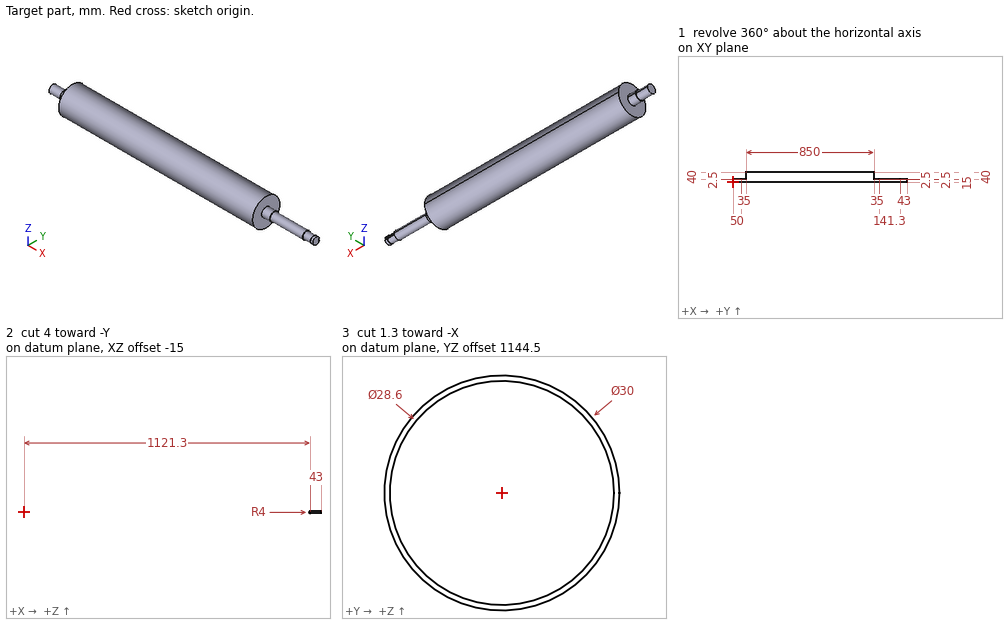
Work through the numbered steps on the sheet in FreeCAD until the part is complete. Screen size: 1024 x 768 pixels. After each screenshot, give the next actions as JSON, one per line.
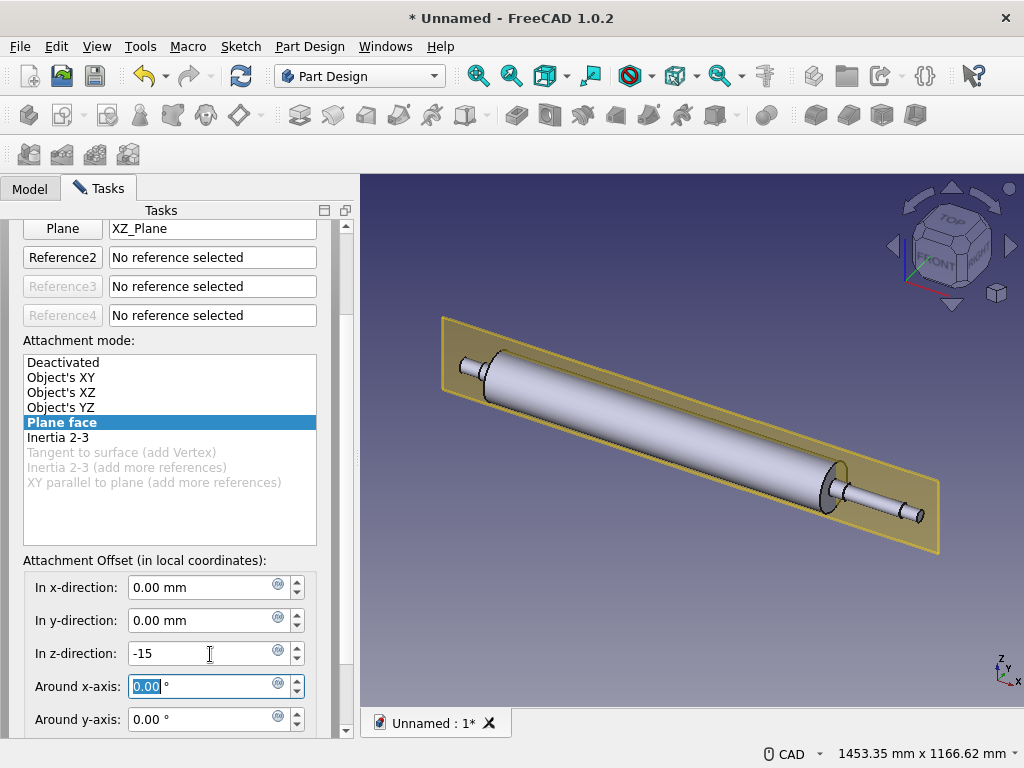
{"action": "scroll", "coordinate": [346, 479], "scroll_direction": "up", "scroll_amount": 3}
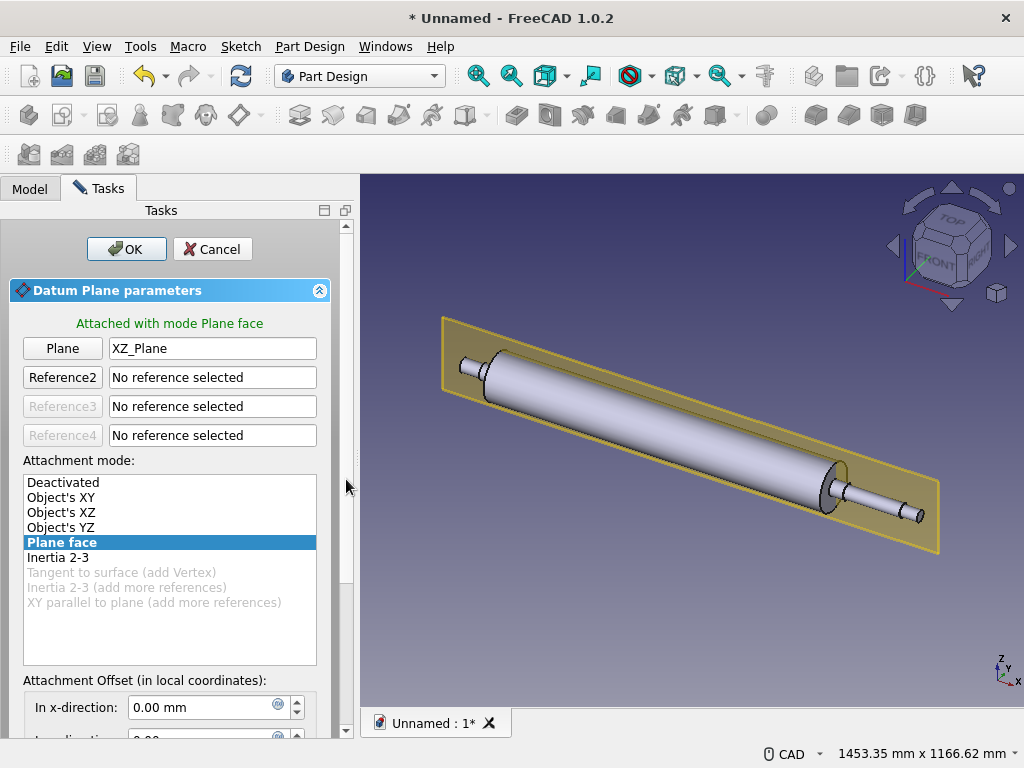
{"action": "left_click", "coordinate": [127, 249]}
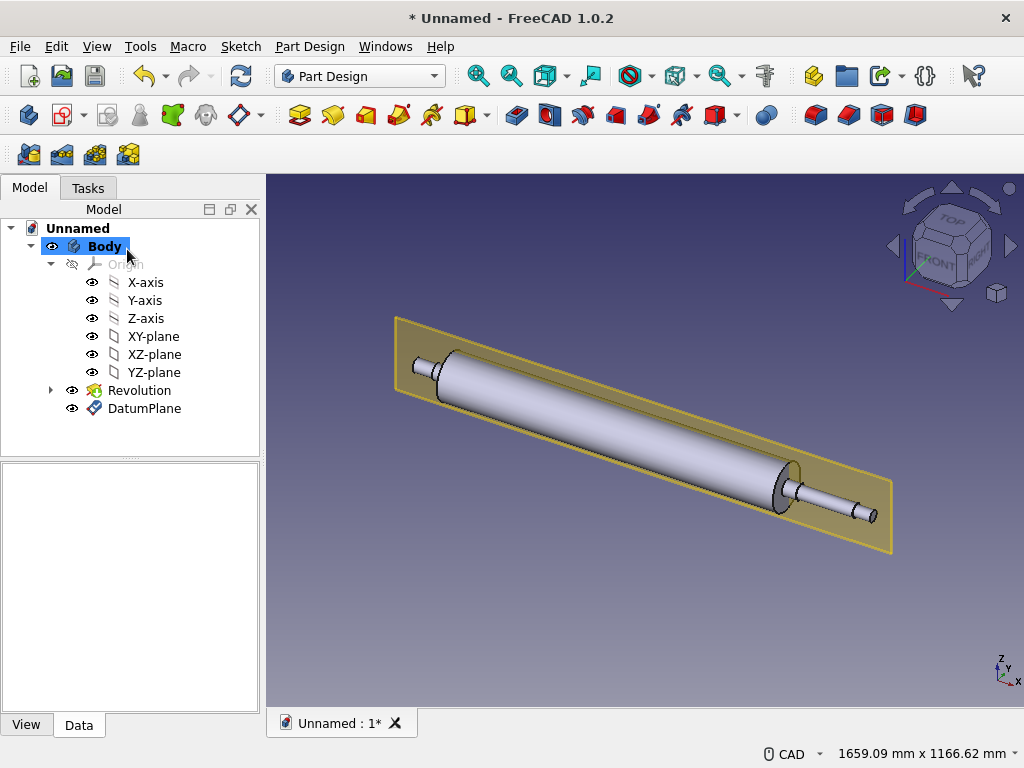
{"action": "left_click", "coordinate": [117, 408]}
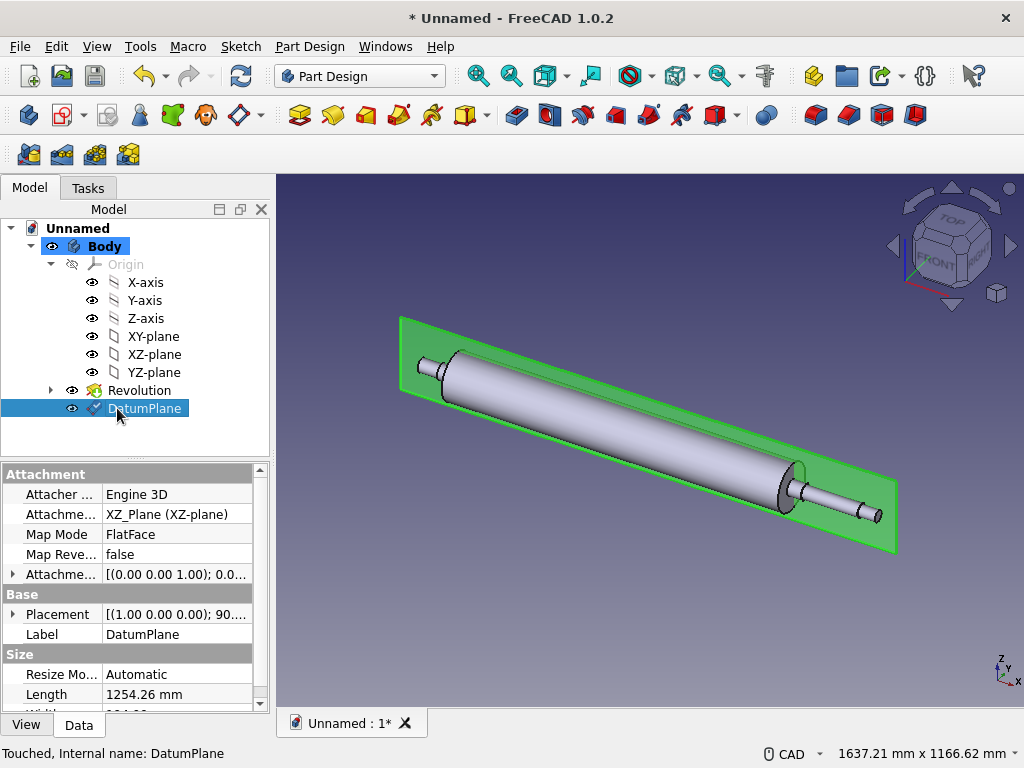
{"action": "left_click", "coordinate": [62, 116]}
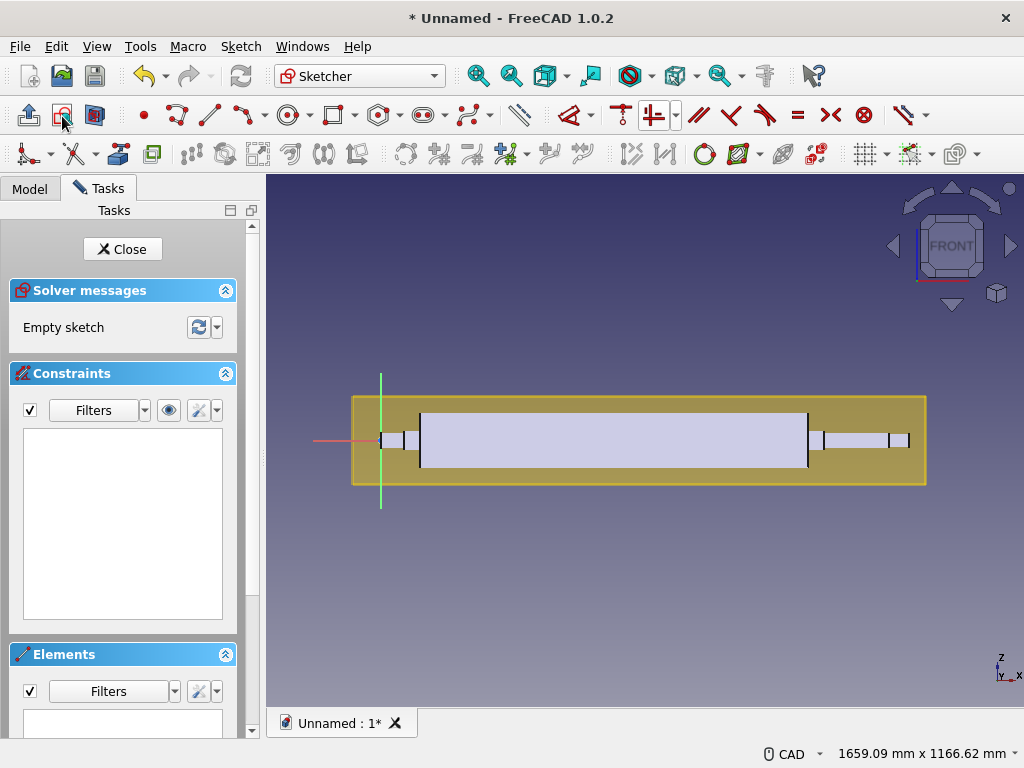
{"action": "left_click", "coordinate": [95, 116]}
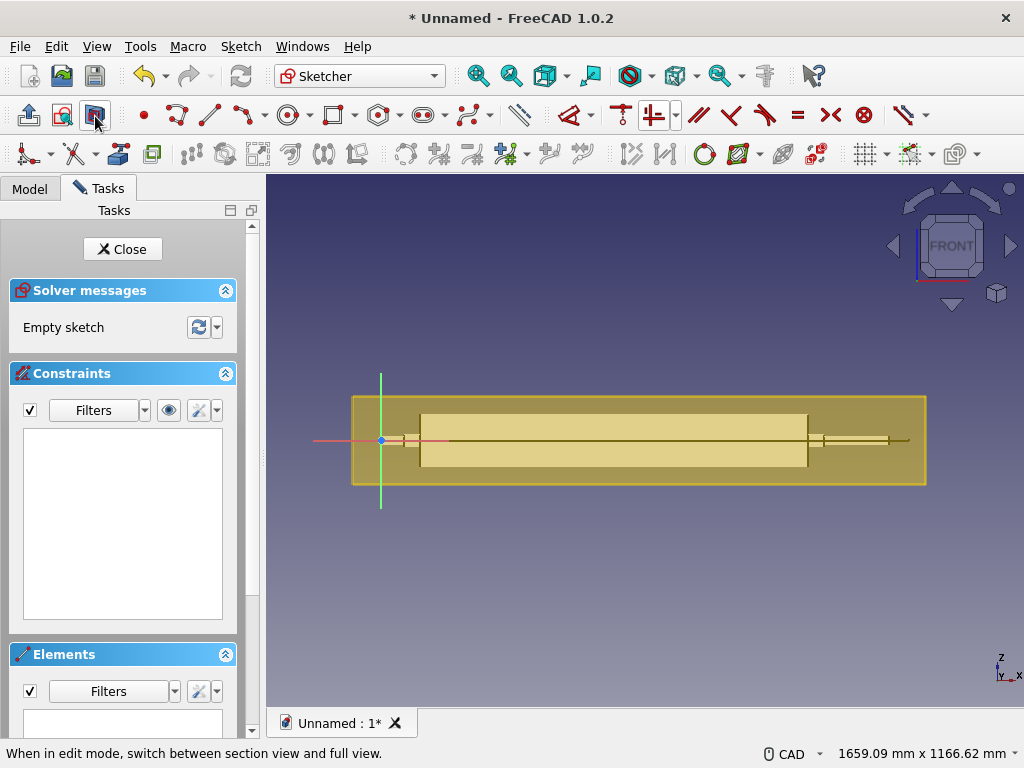
{"action": "scroll", "coordinate": [576, 440], "scroll_direction": "down", "scroll_amount": 5}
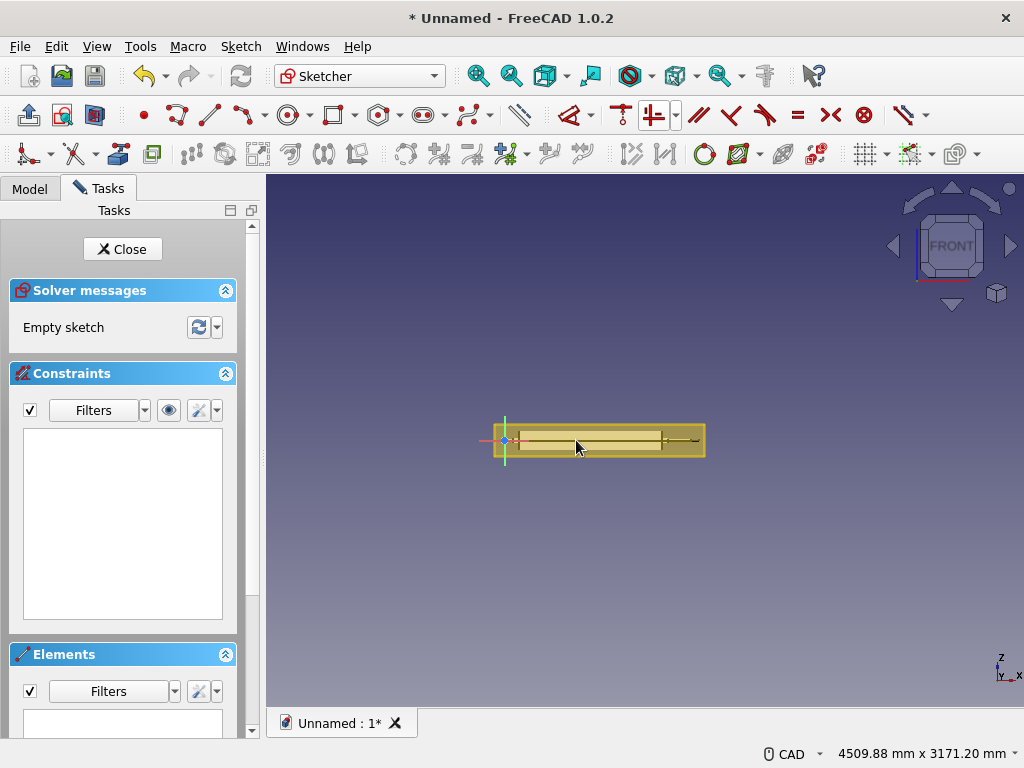
{"action": "scroll", "coordinate": [703, 441], "scroll_direction": "up", "scroll_amount": 15}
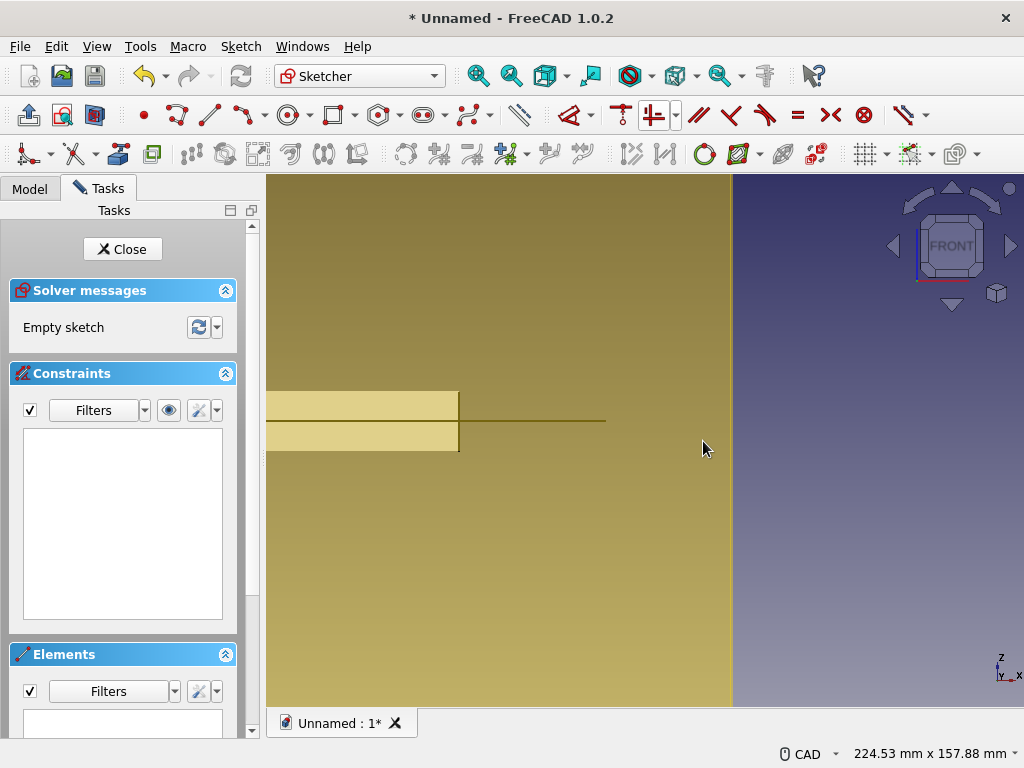
{"action": "scroll", "coordinate": [549, 410], "scroll_direction": "up", "scroll_amount": 5}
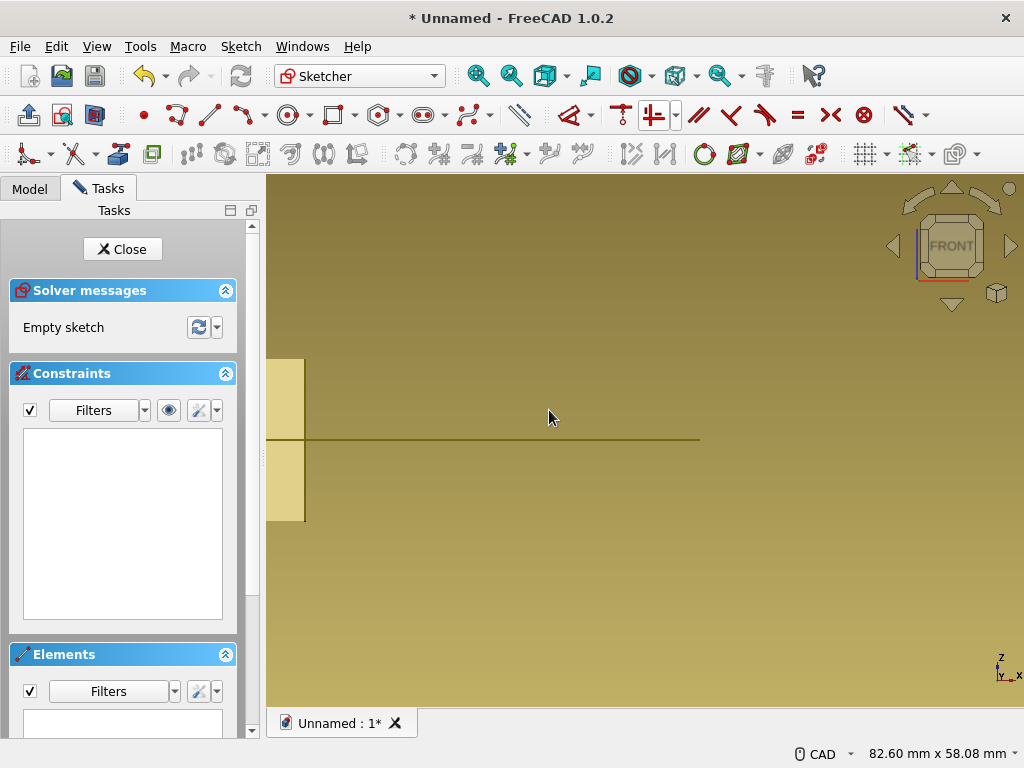
{"action": "left_click", "coordinate": [177, 116]}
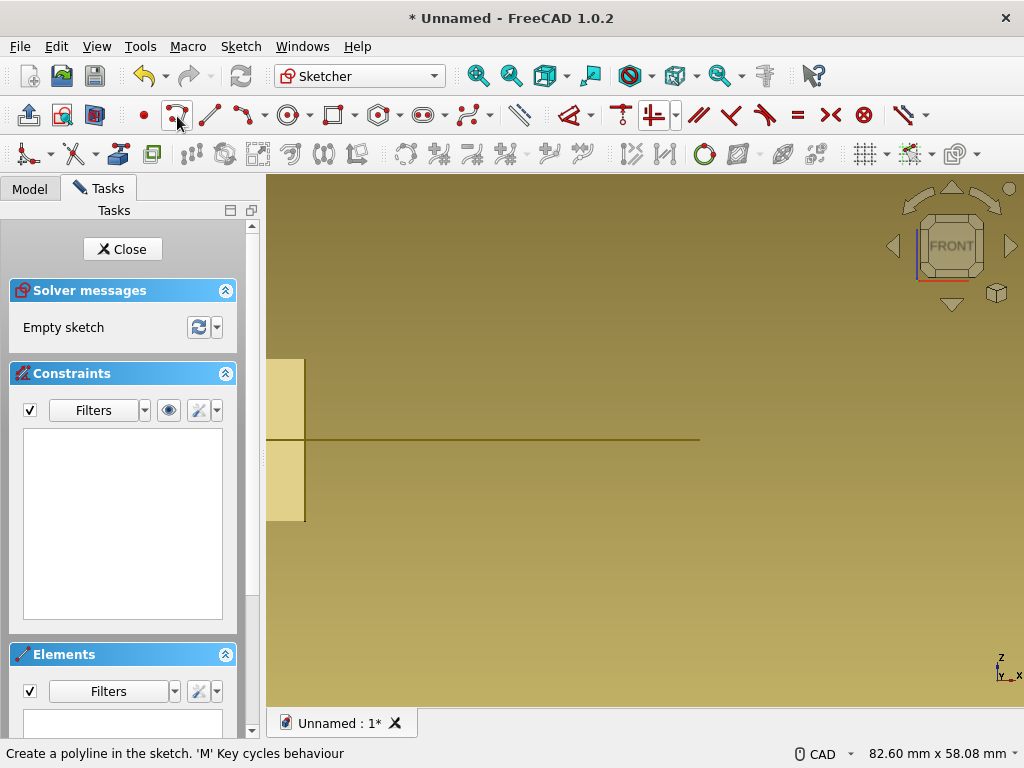
{"action": "left_click", "coordinate": [397, 403]}
{"action": "left_click", "coordinate": [791, 403]}
{"action": "left_click", "coordinate": [791, 477]}
{"action": "left_click", "coordinate": [397, 477]}
{"action": "right_click", "coordinate": [397, 477]}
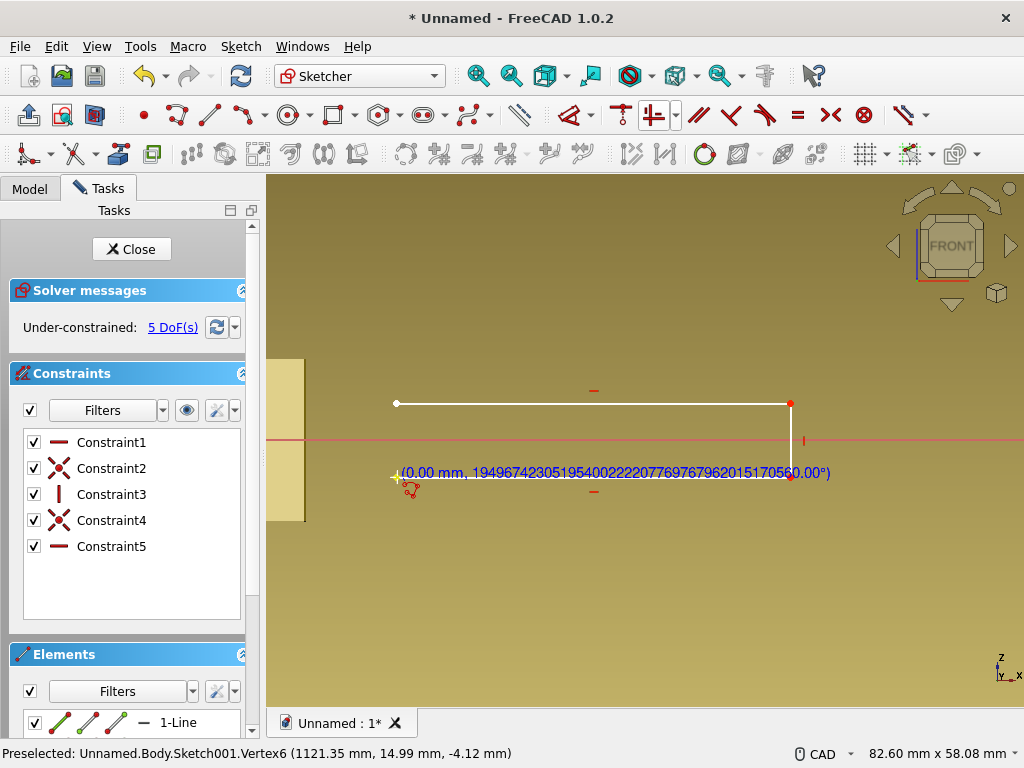
{"action": "key", "text": "g 3 a"}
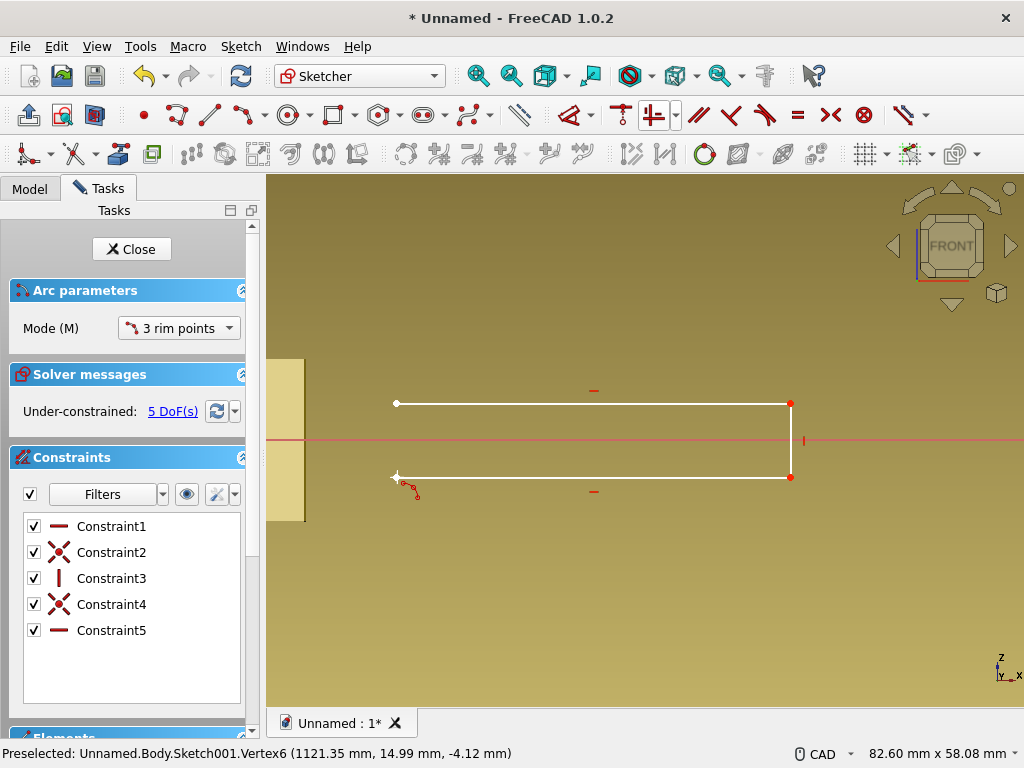
{"action": "left_click", "coordinate": [397, 478]}
{"action": "left_click", "coordinate": [397, 404]}
{"action": "left_click", "coordinate": [367, 419]}
{"action": "key", "text": "Escape"}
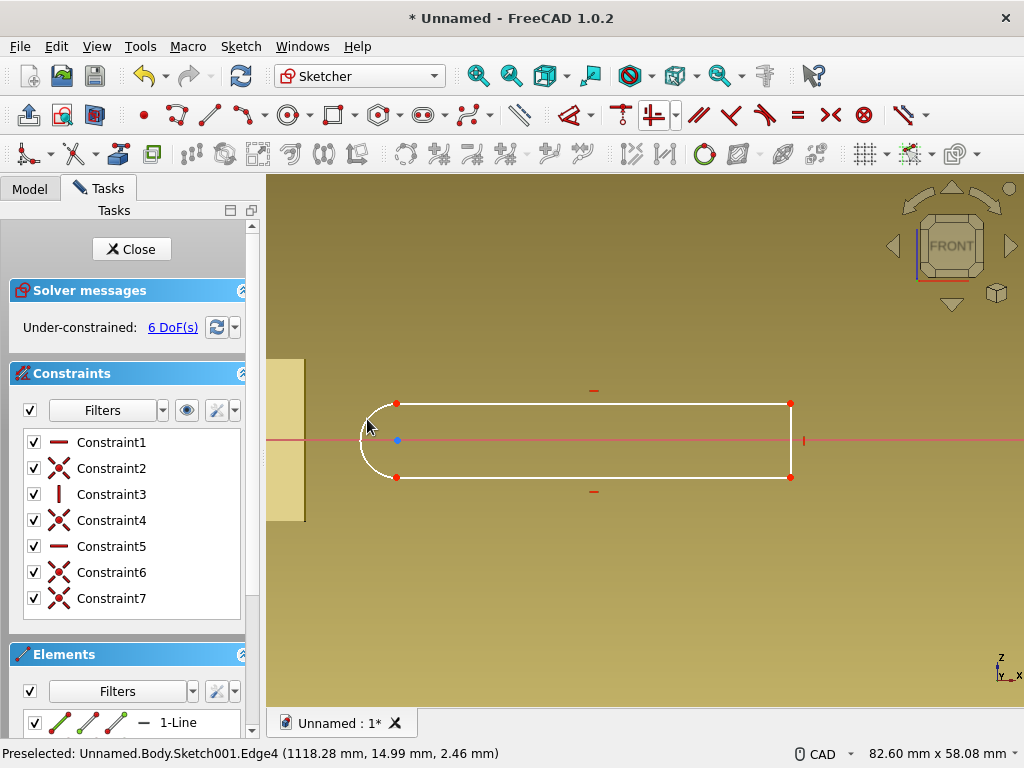
{"action": "left_click", "coordinate": [515, 404]}